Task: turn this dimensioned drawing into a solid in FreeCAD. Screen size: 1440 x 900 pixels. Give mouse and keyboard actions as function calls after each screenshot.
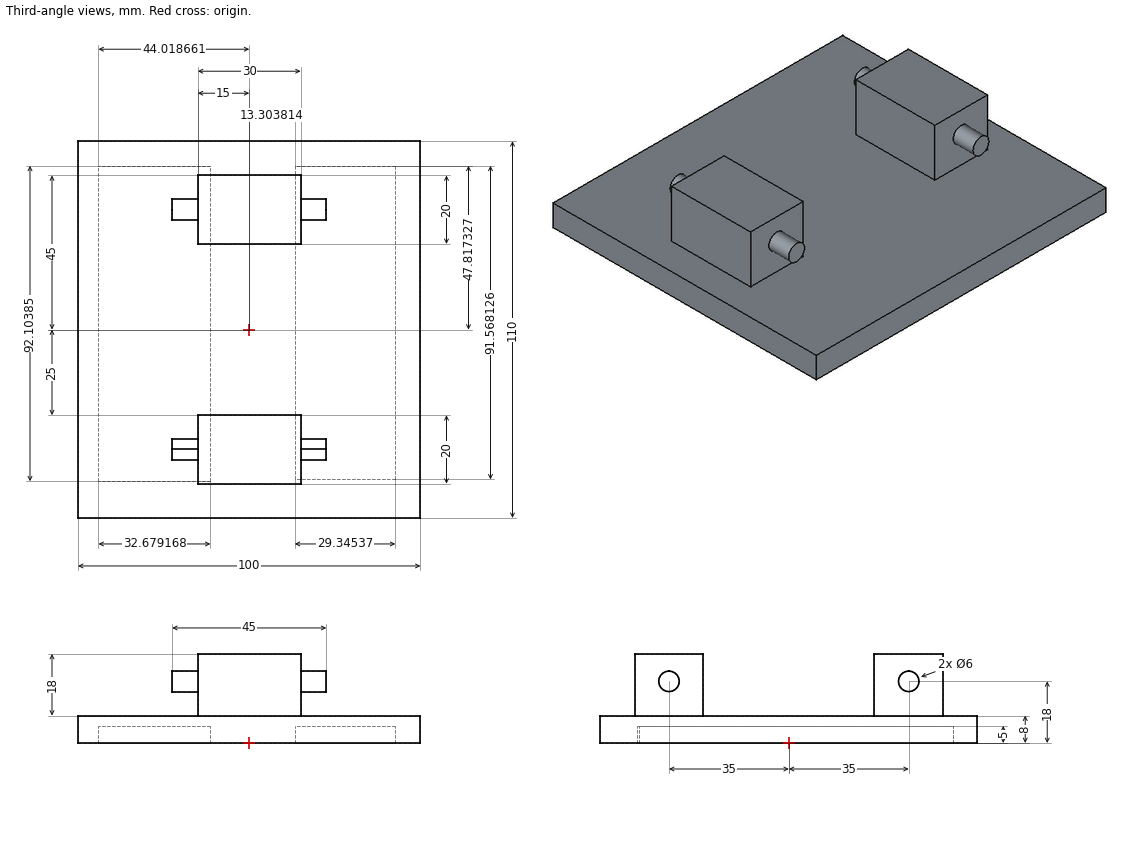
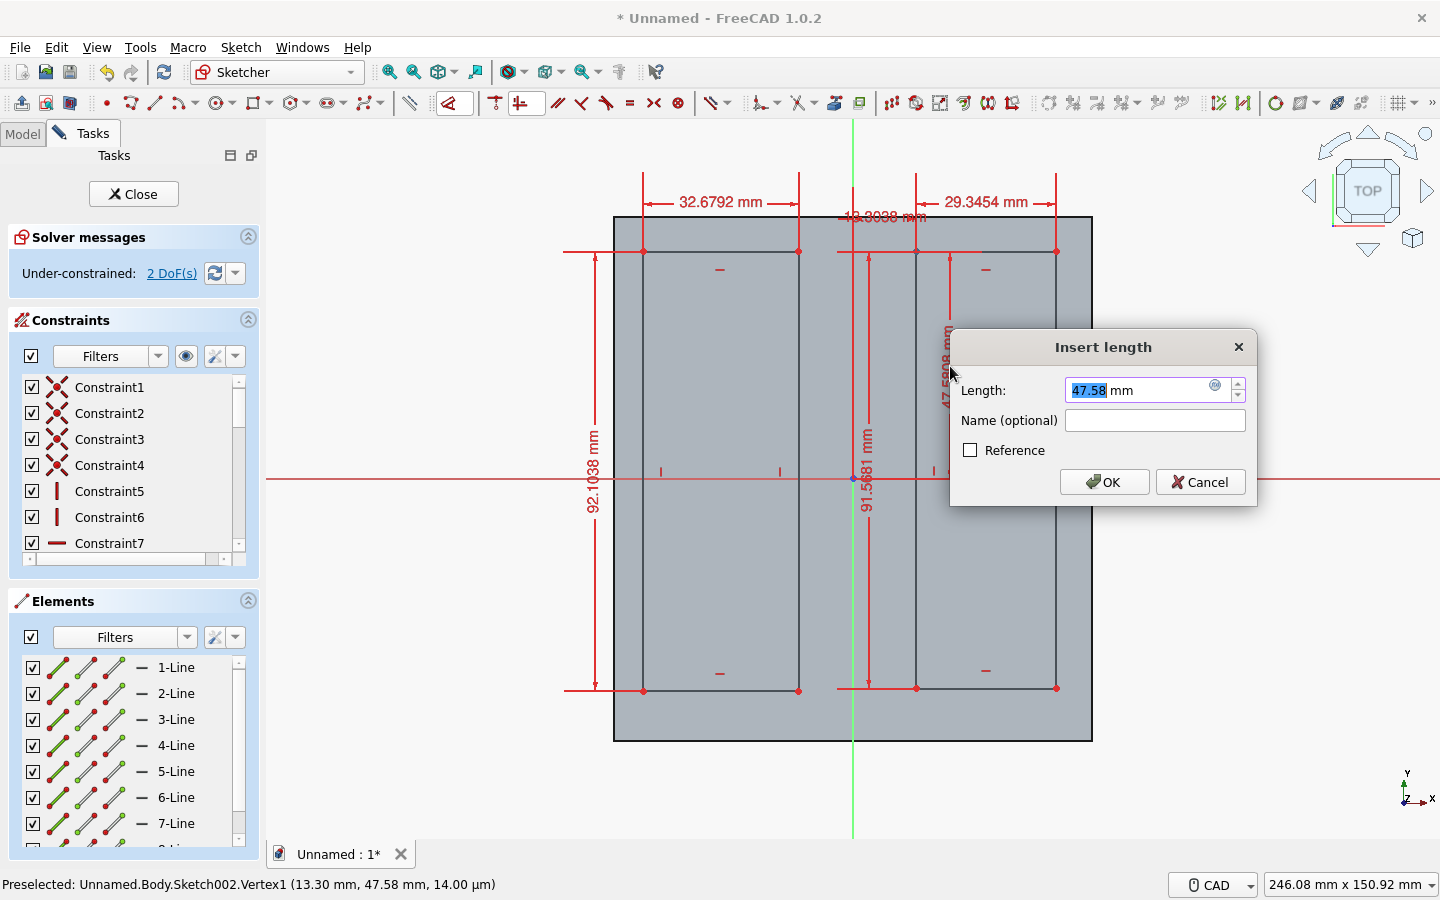
text(47.817327)
key(Return)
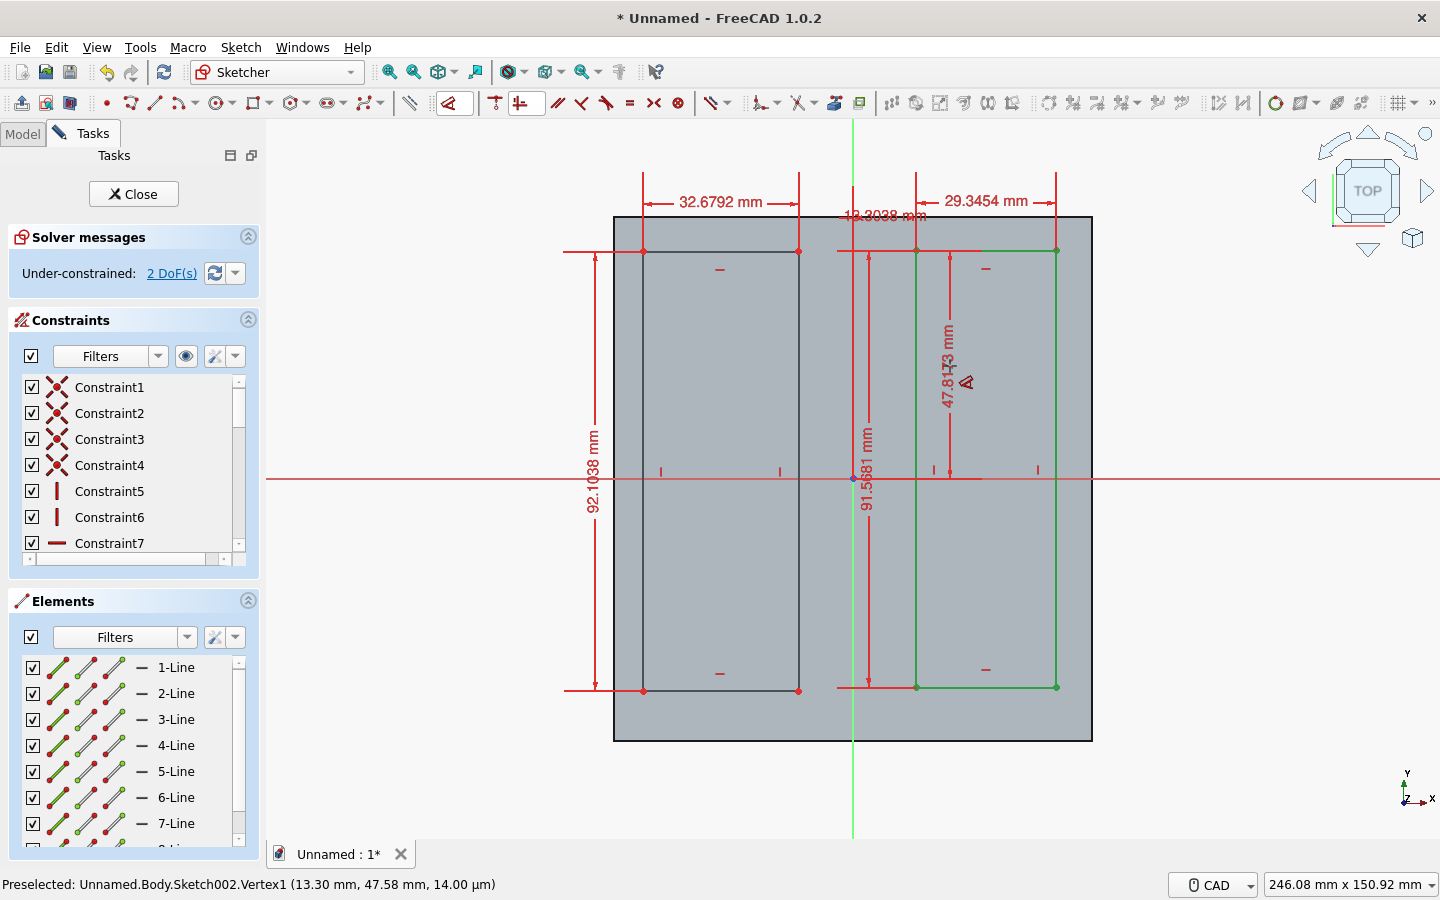
click(643, 252)
click(748, 218)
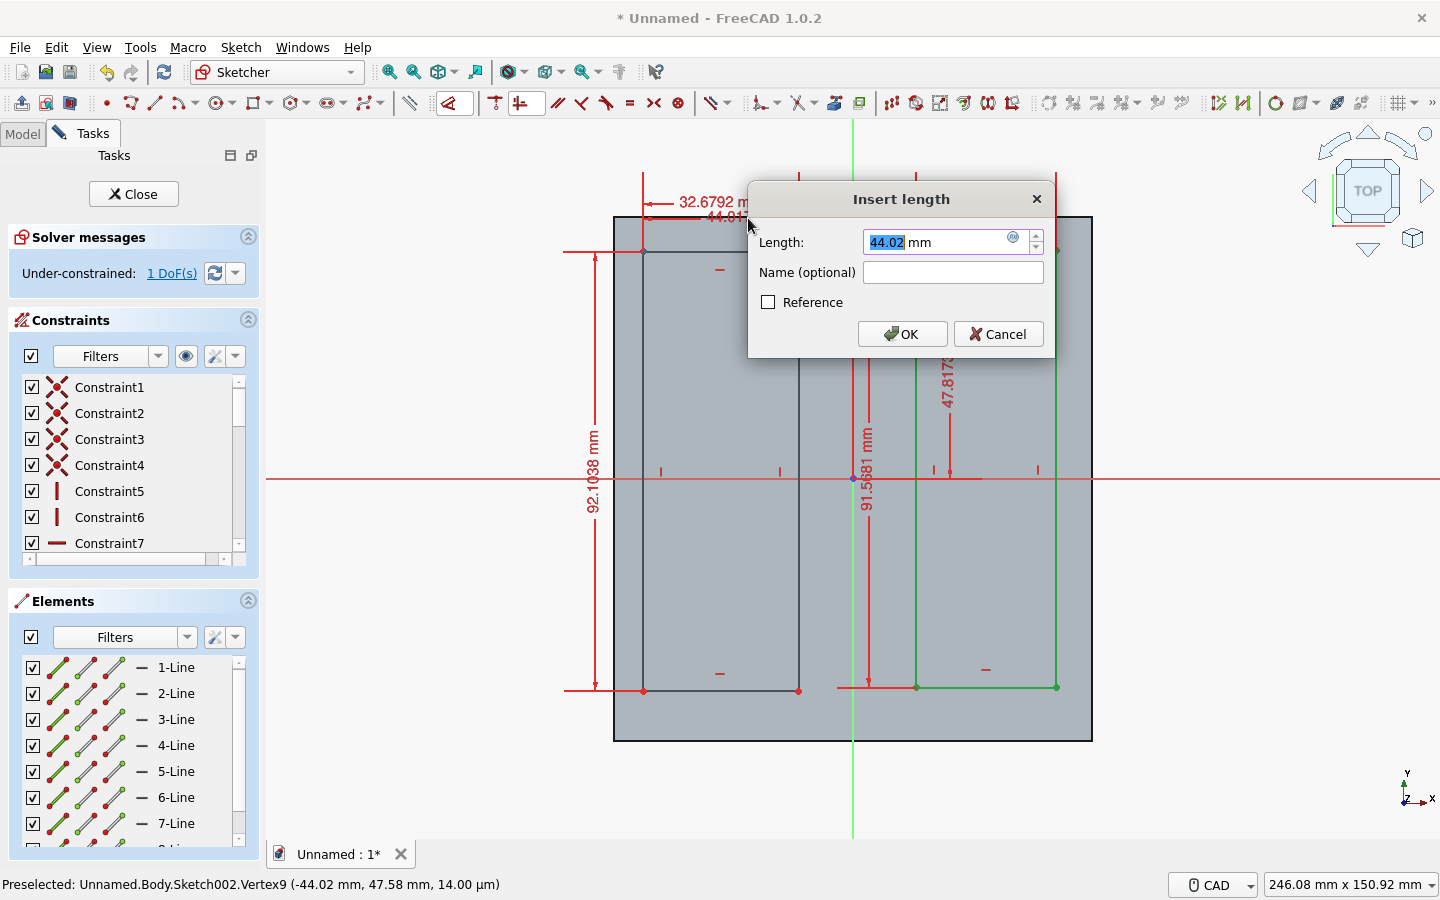
text(44.018661)
key(Return)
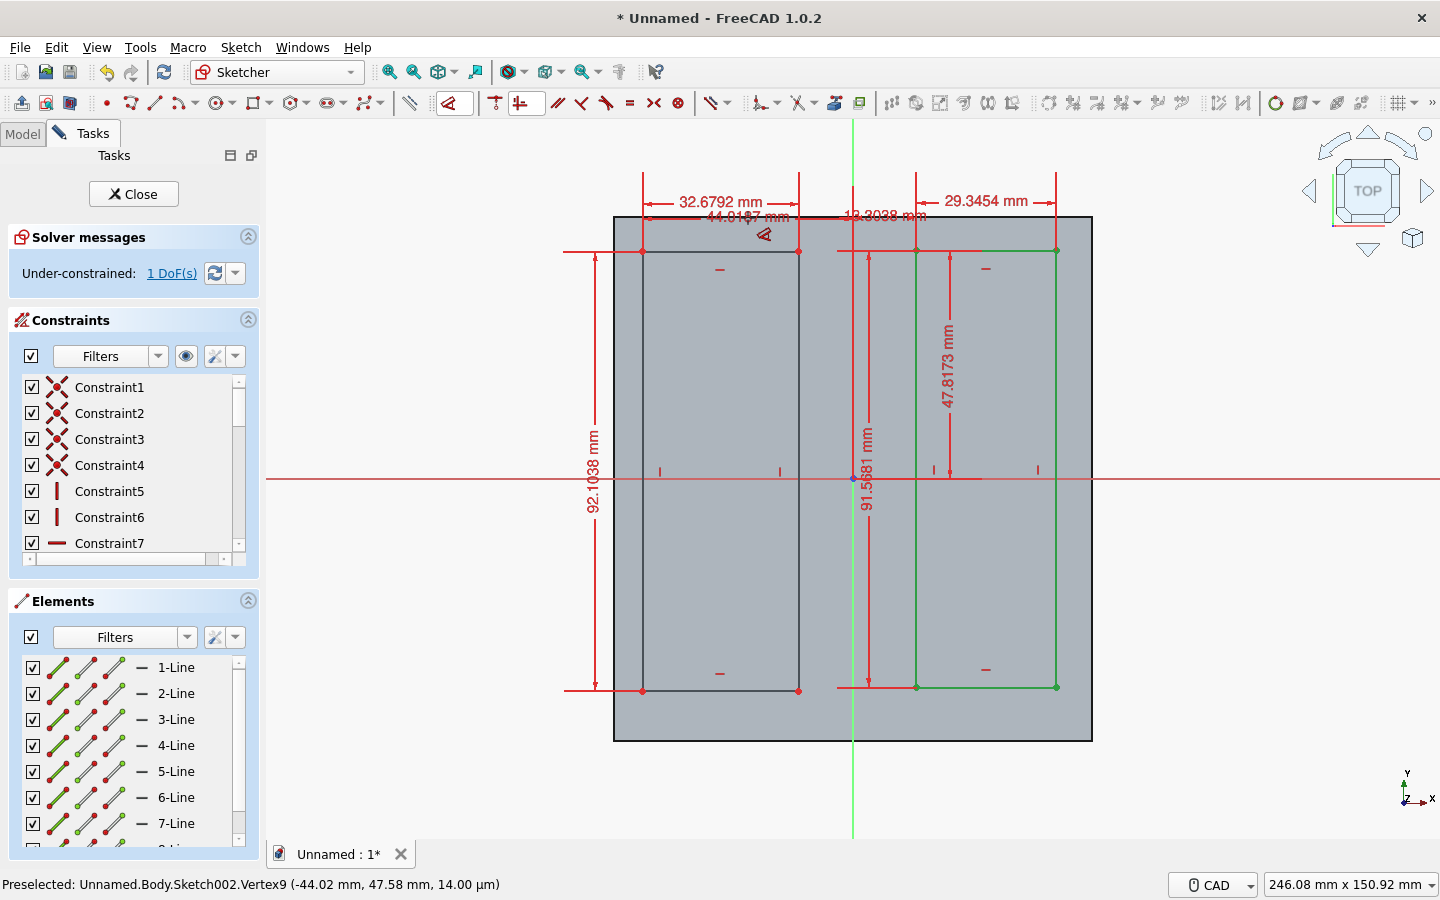
click(643, 252)
click(609, 366)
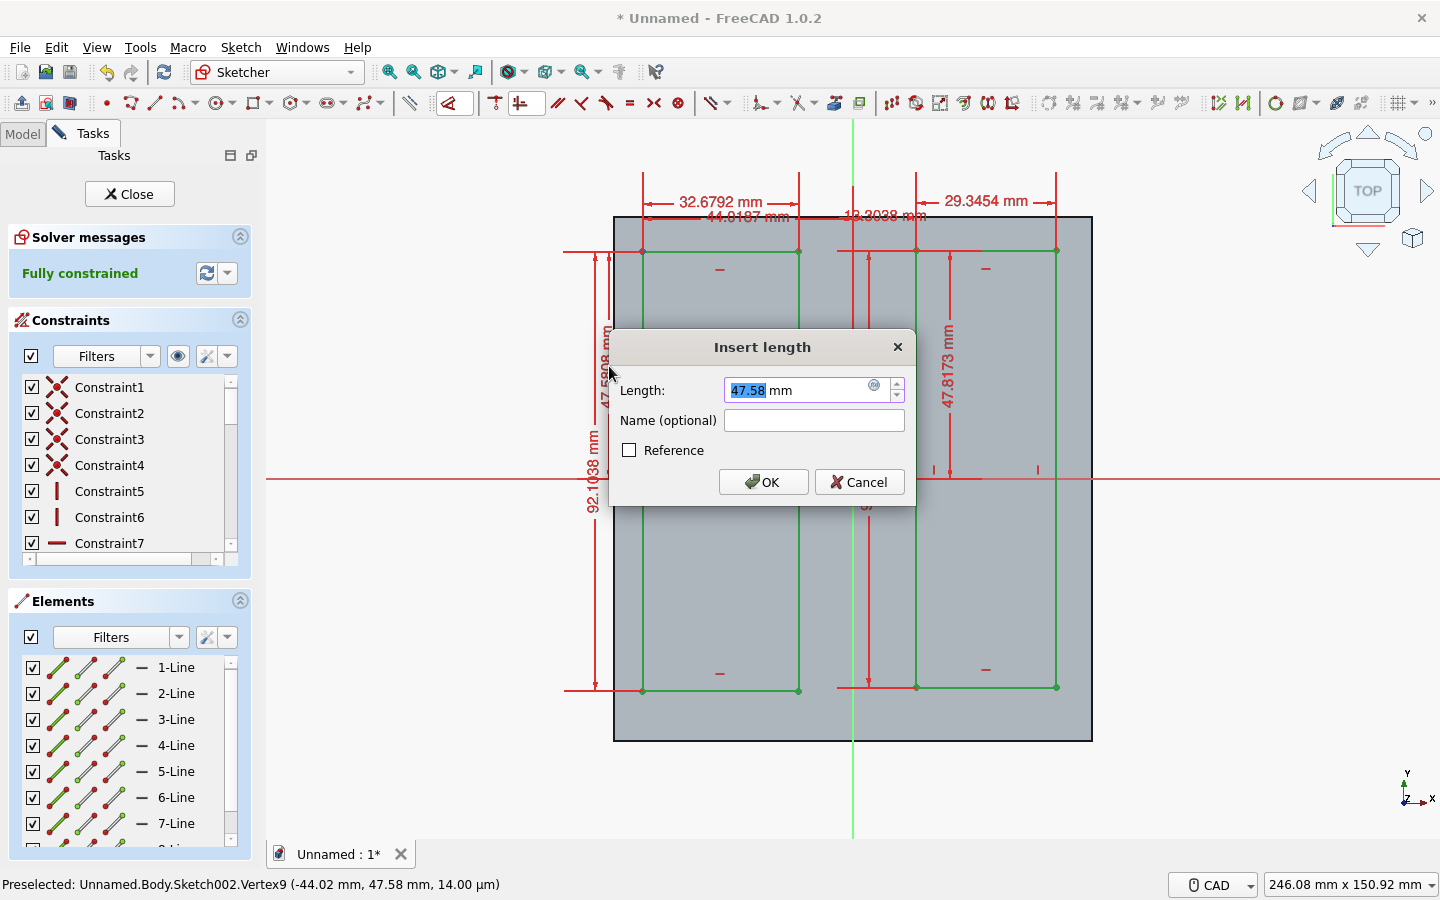
text(47.817327)
key(Return)
key(Escape)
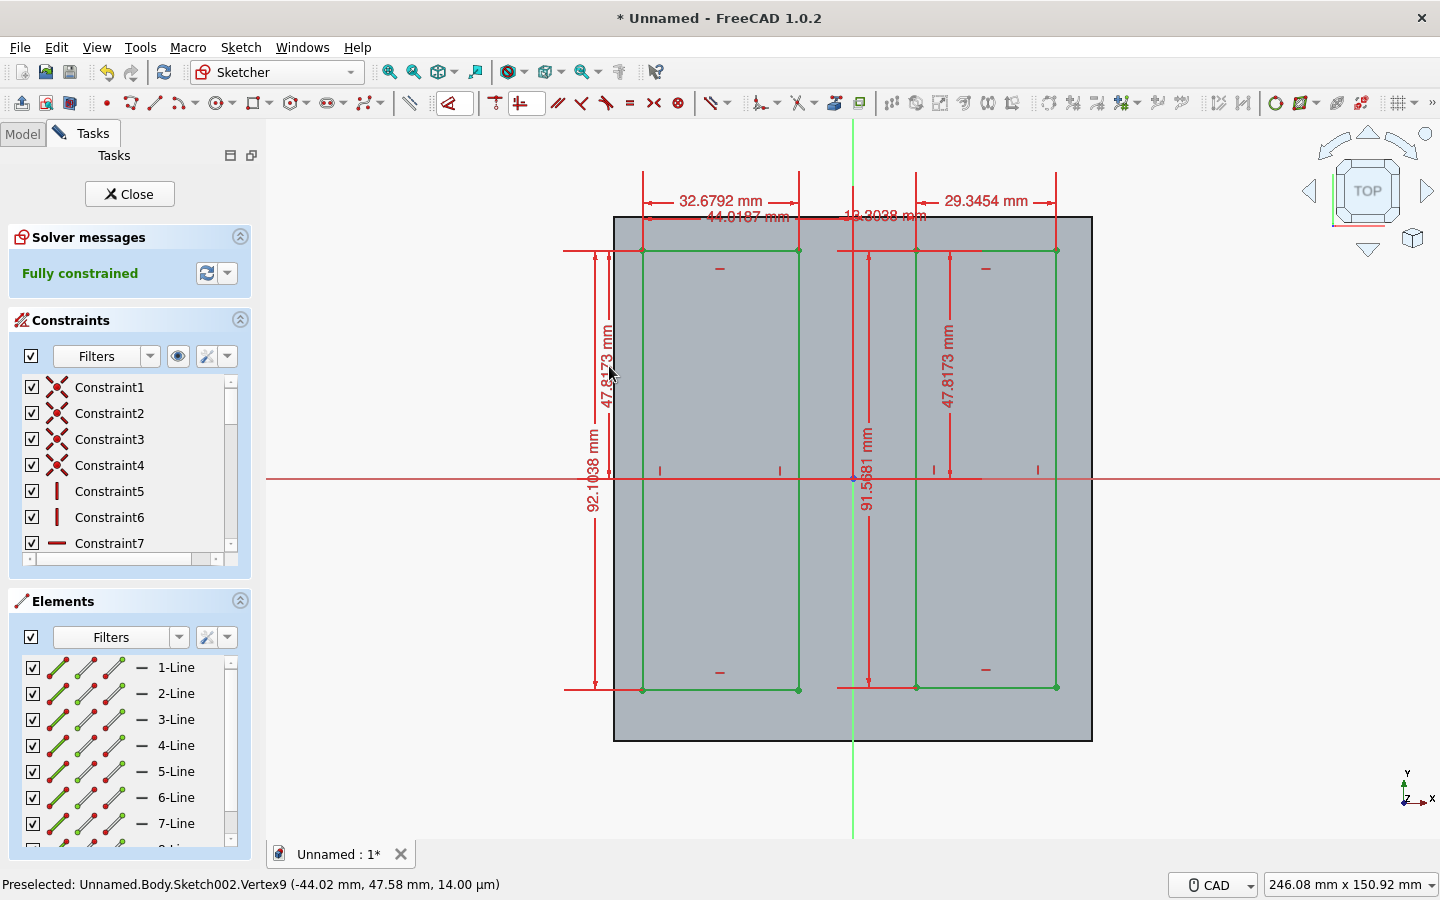
click(130, 194)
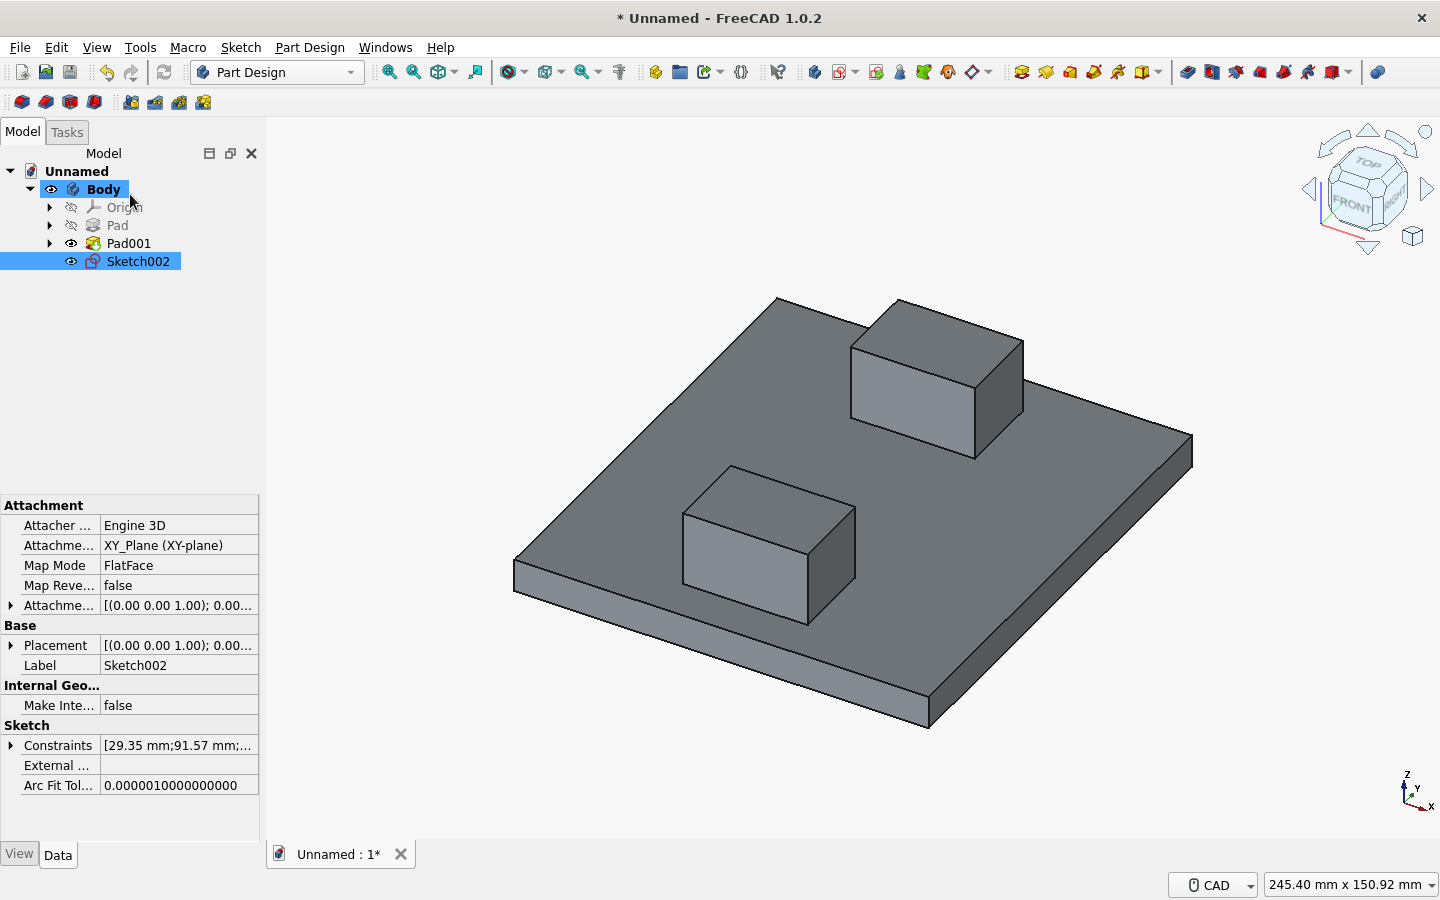
click(1188, 72)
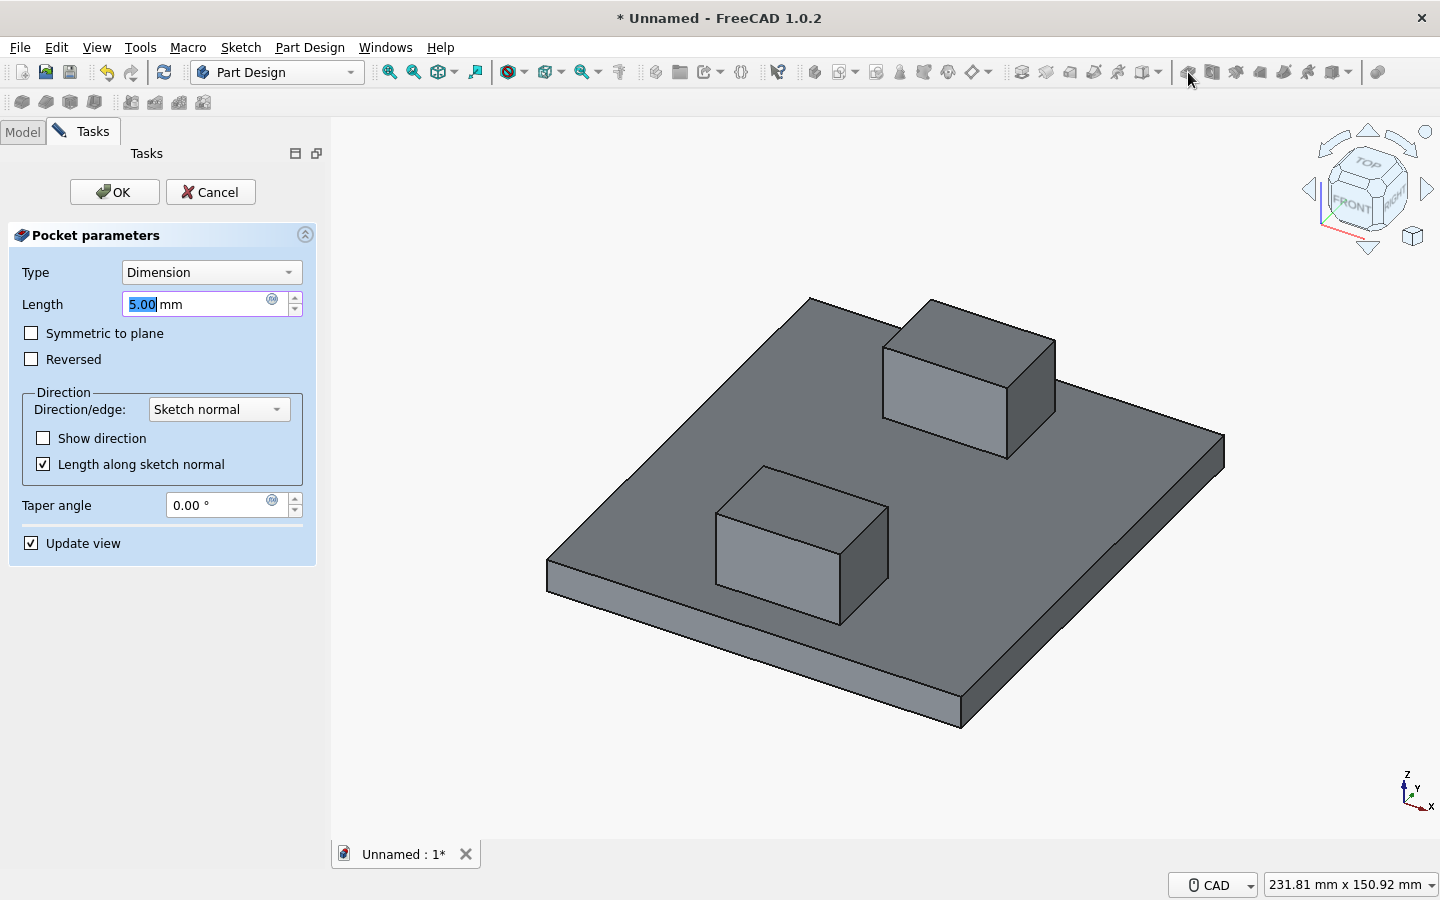
text(5)
key(Tab)